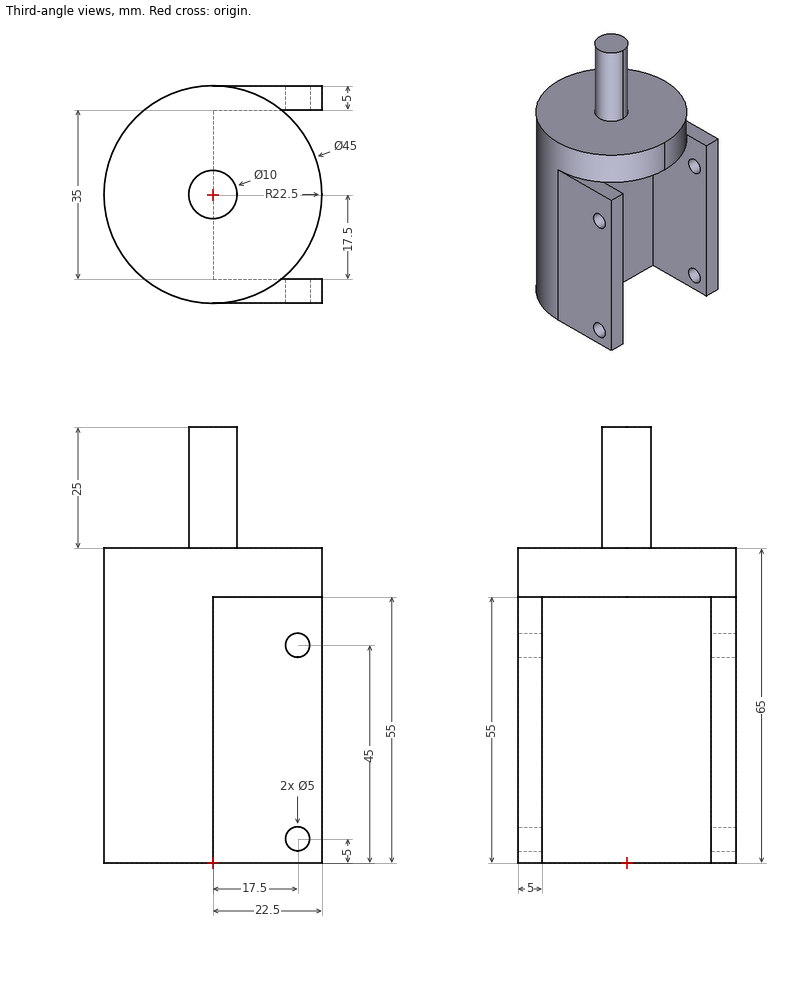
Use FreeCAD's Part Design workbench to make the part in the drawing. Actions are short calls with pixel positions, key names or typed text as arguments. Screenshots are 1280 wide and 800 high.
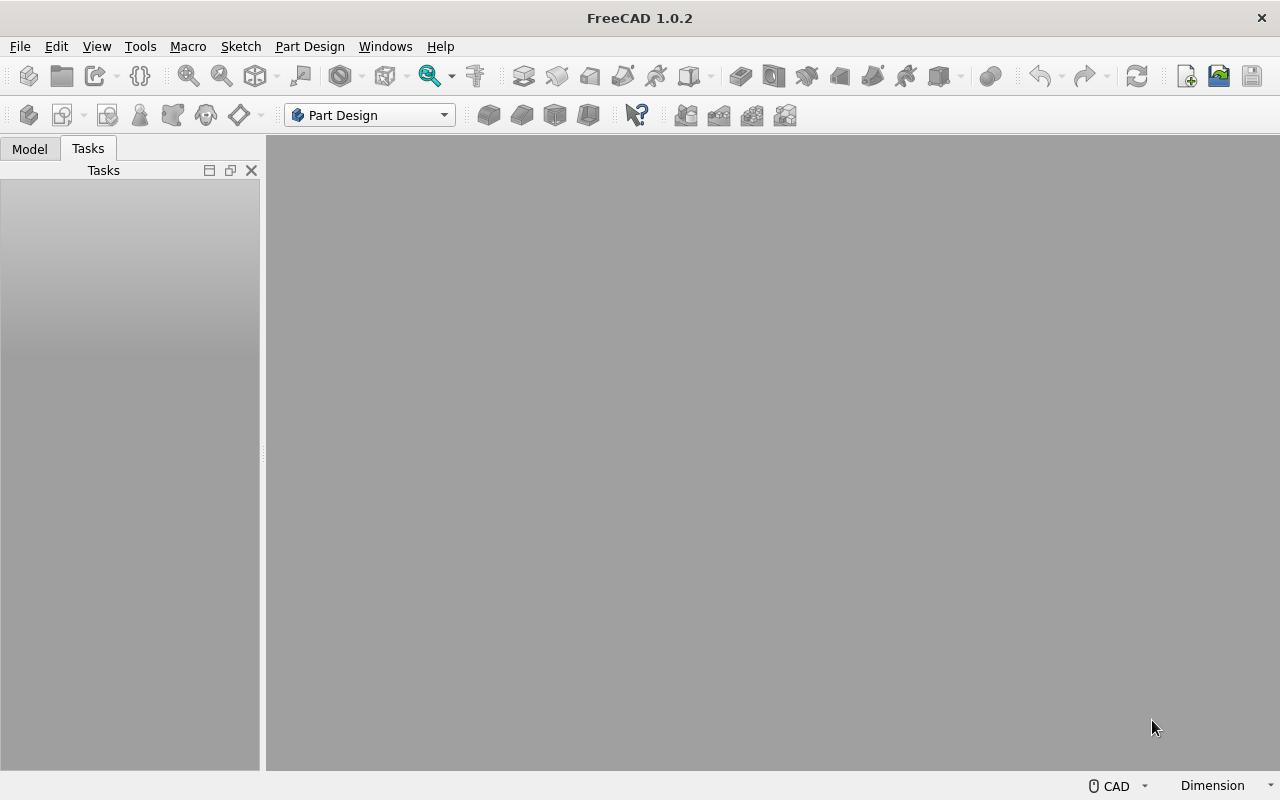
click(1186, 76)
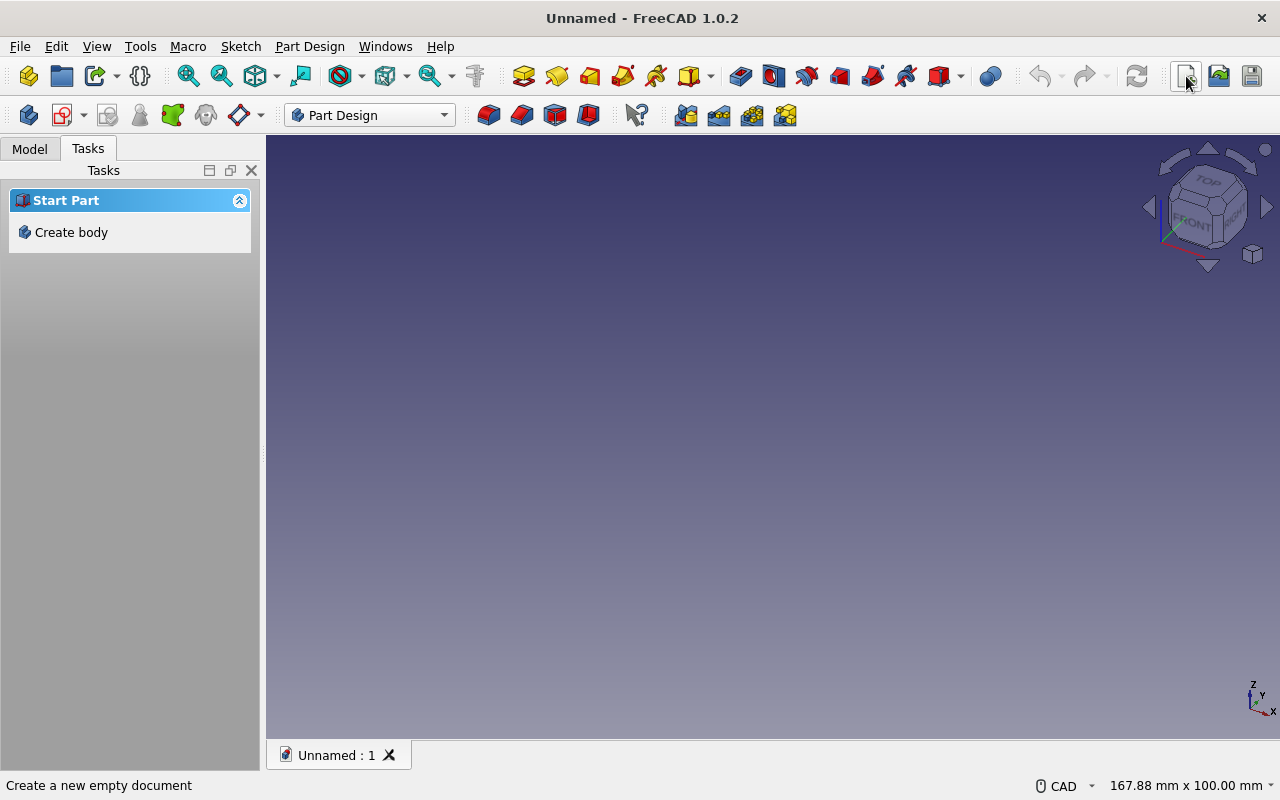
click(62, 116)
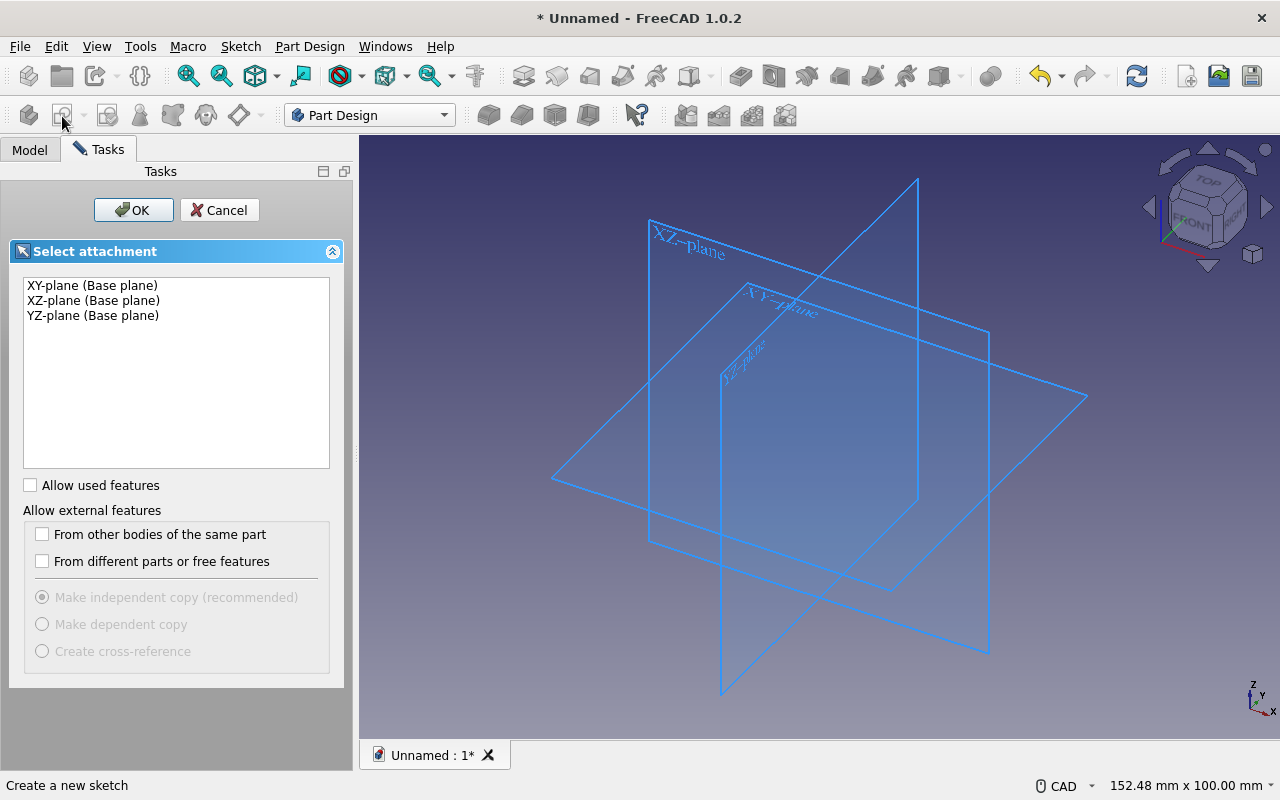
click(84, 286)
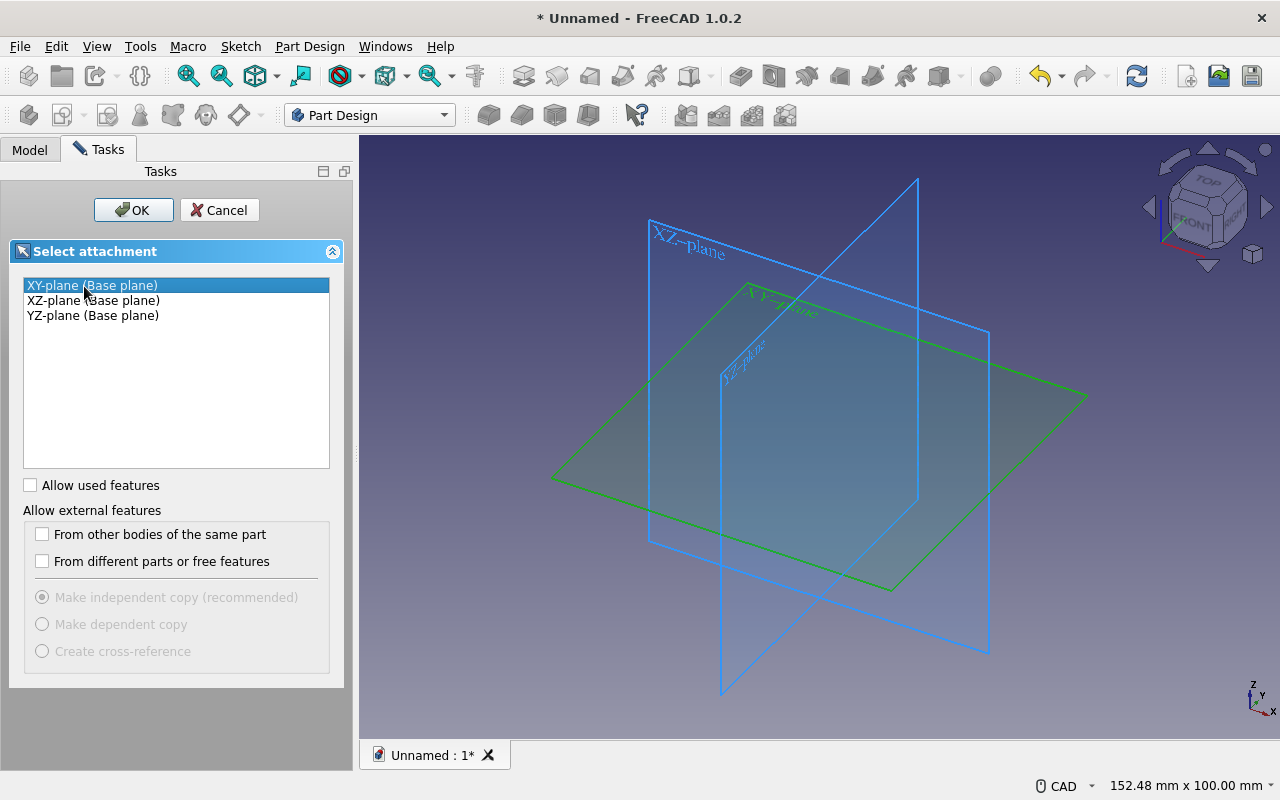
click(134, 210)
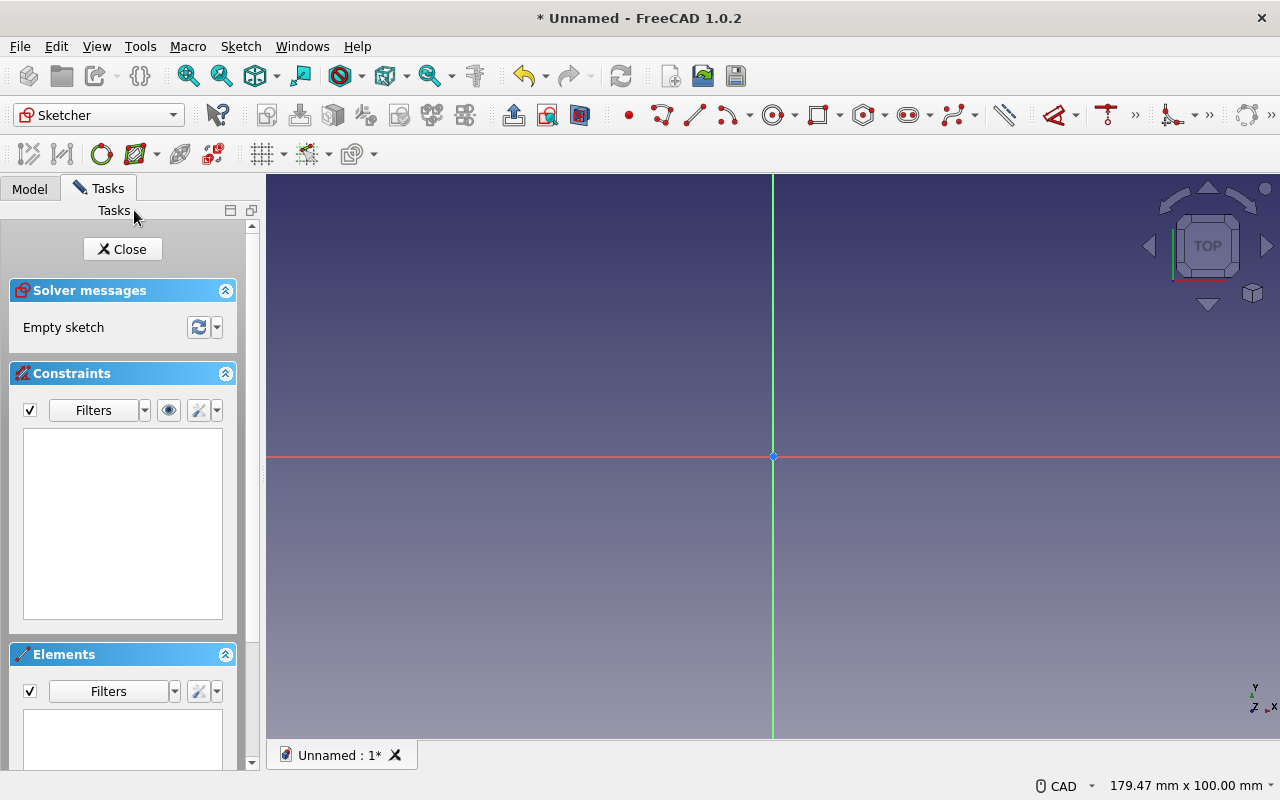
scroll(912, 456, up, 2)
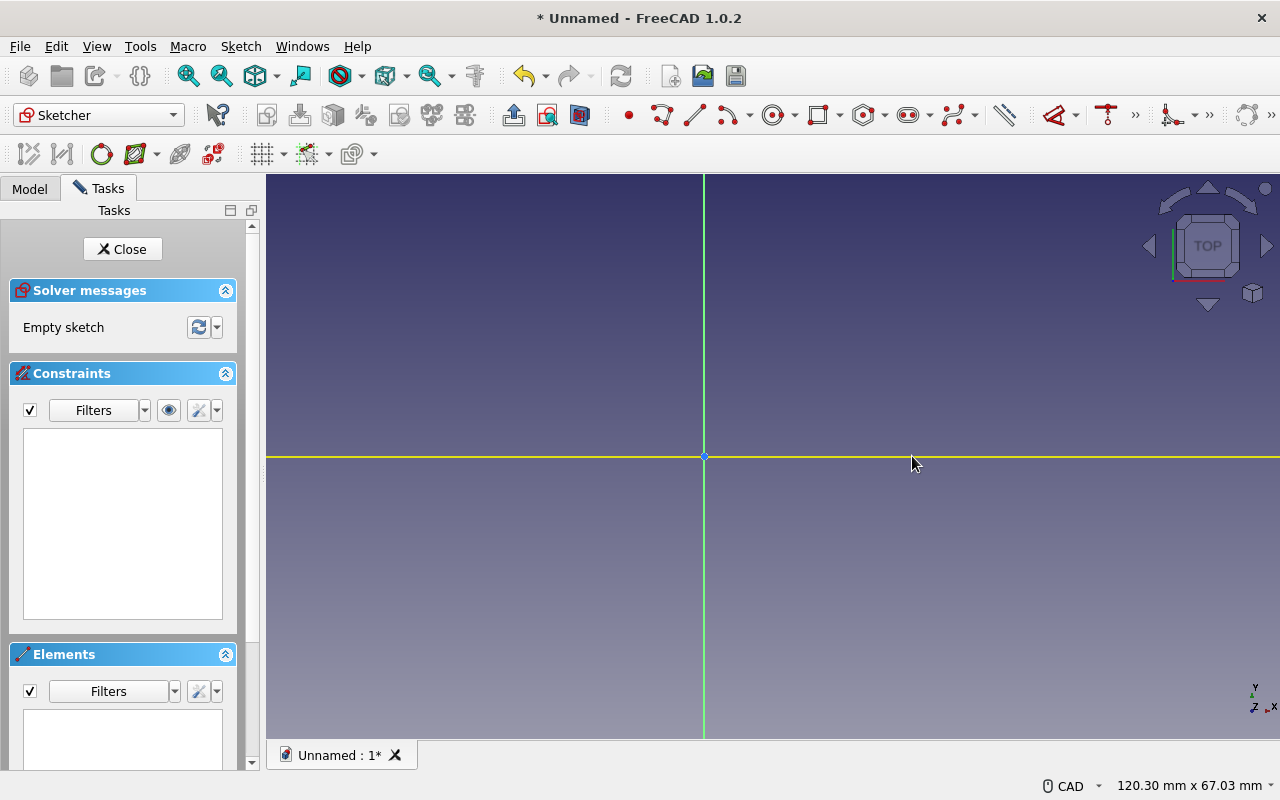
click(772, 116)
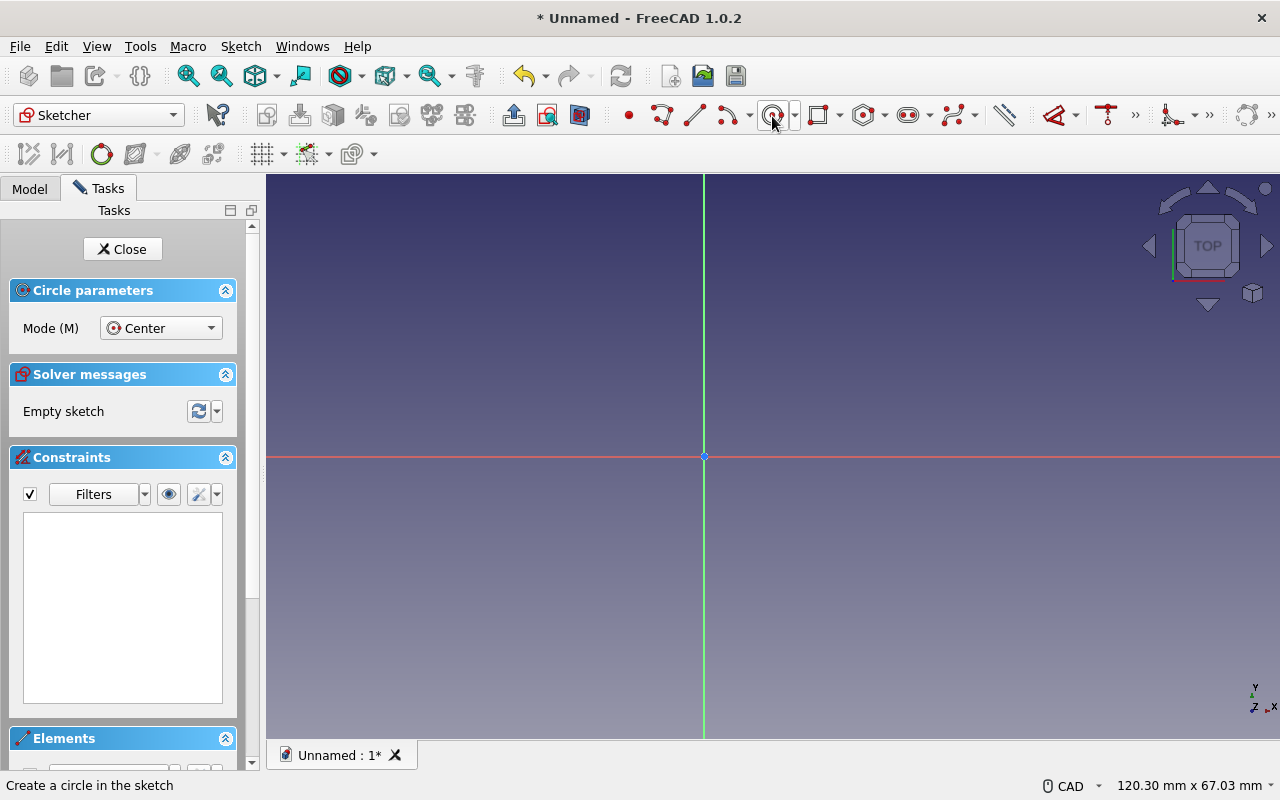
click(704, 456)
click(838, 322)
key(Escape)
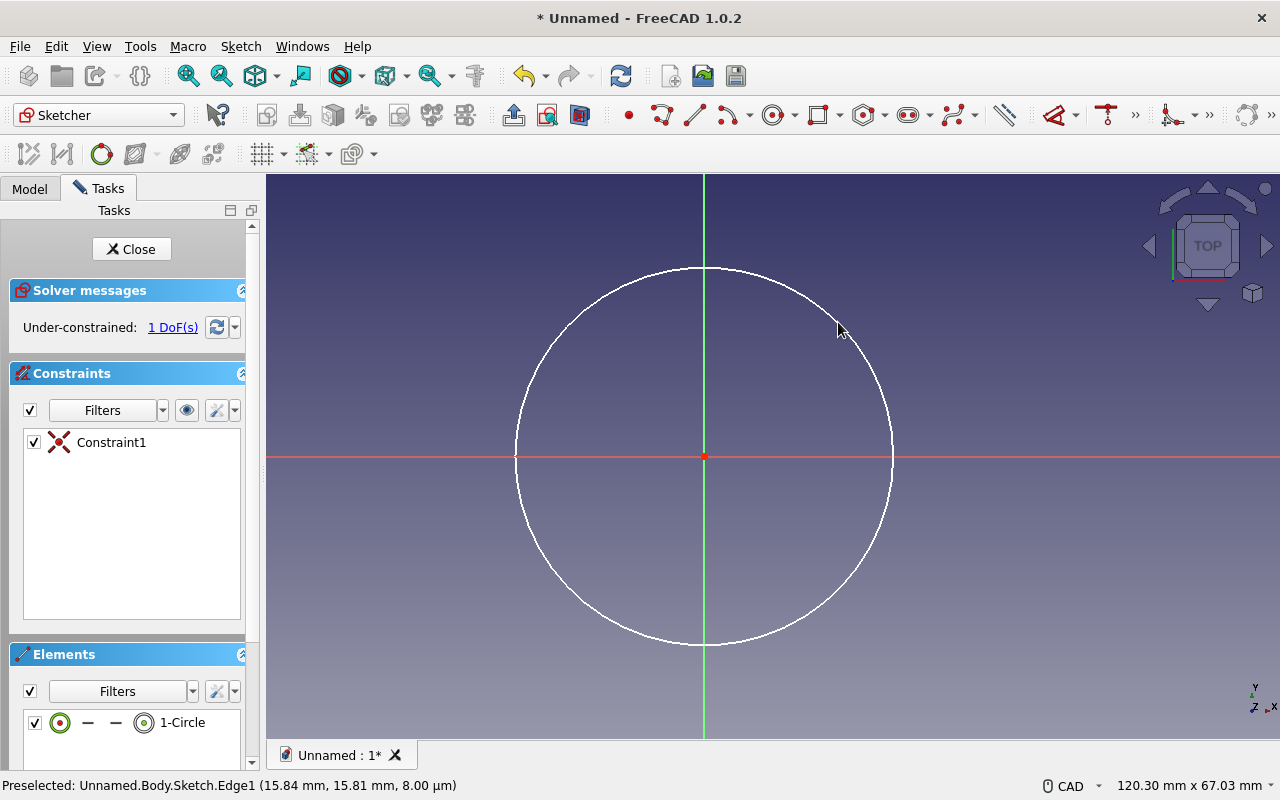
click(1054, 116)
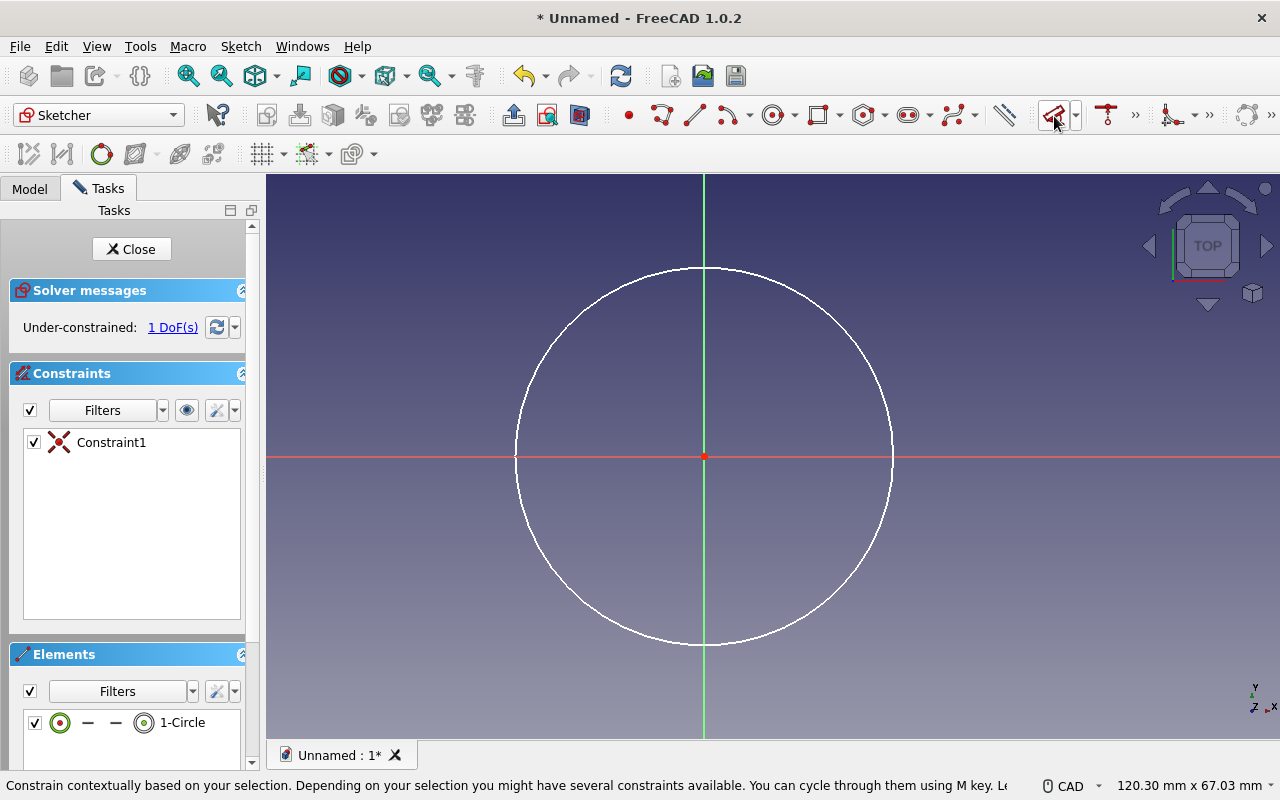
click(837, 322)
click(859, 299)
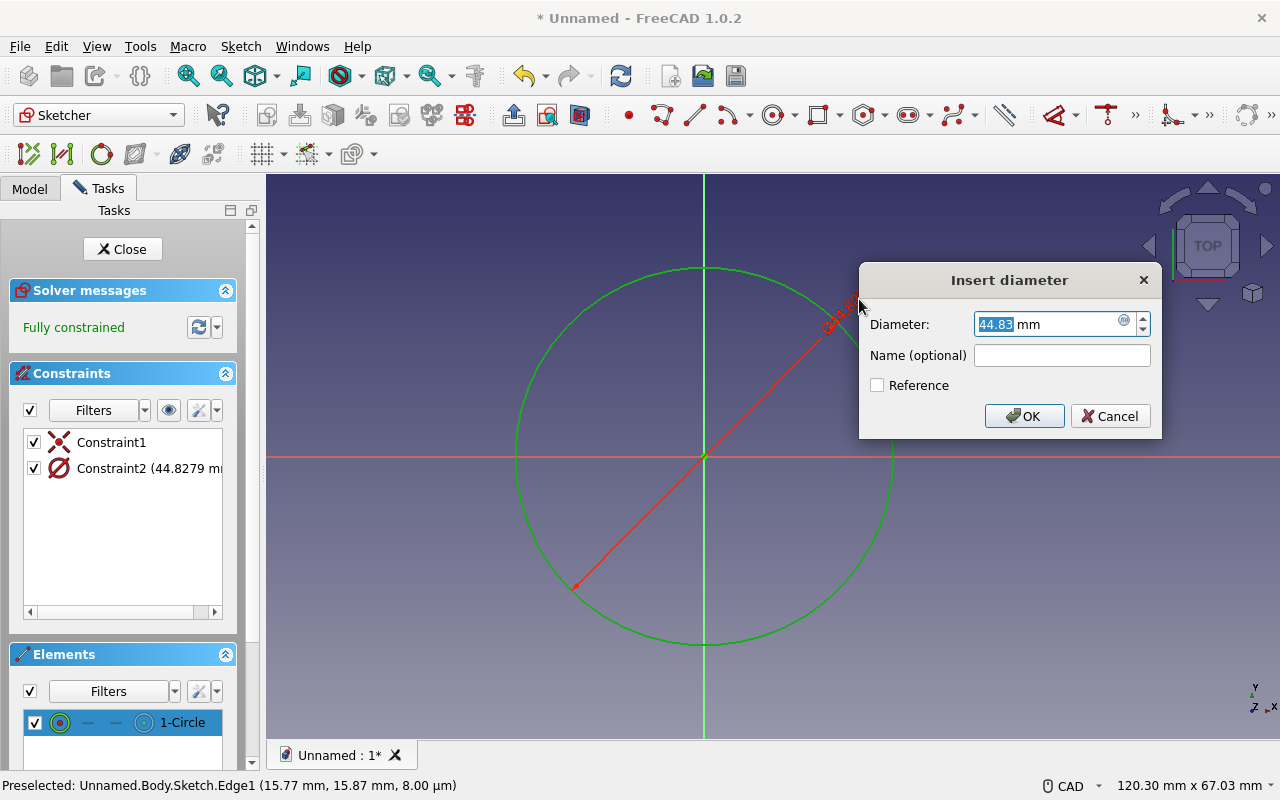
text(45)
key(Return)
key(Escape)